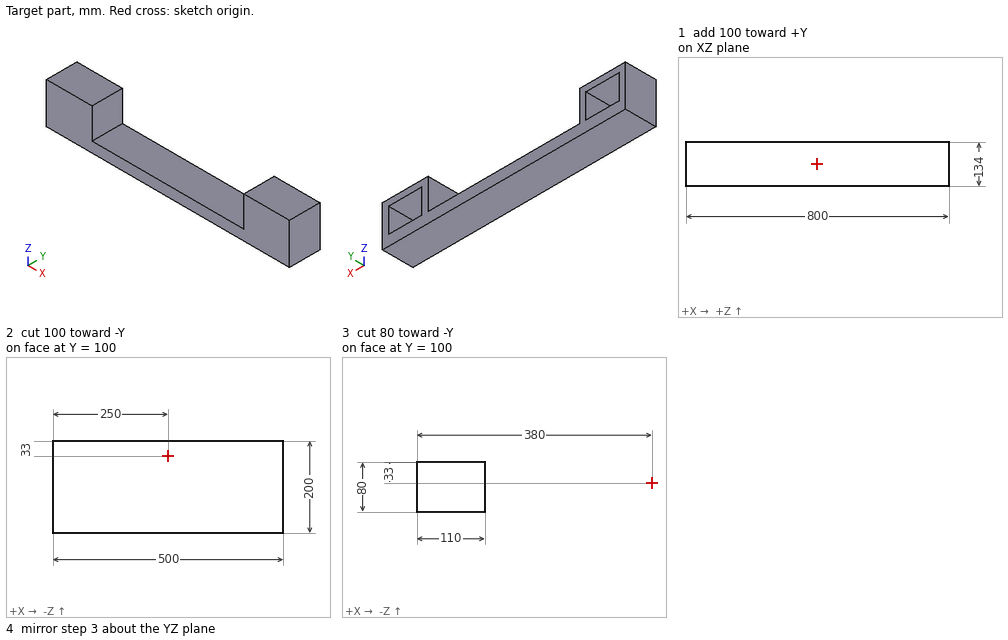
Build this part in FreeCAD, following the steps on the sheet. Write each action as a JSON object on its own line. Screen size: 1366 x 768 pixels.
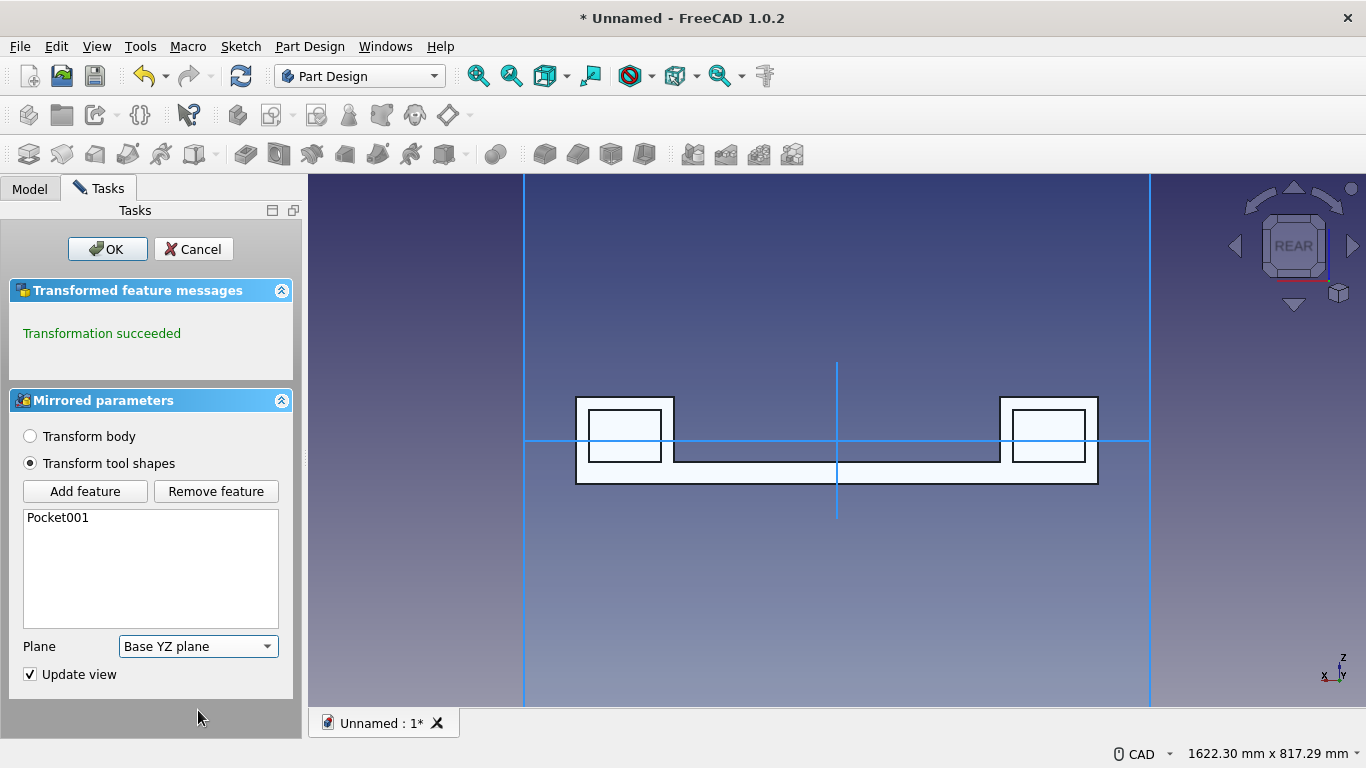
{"action": "left_click", "coordinate": [108, 249]}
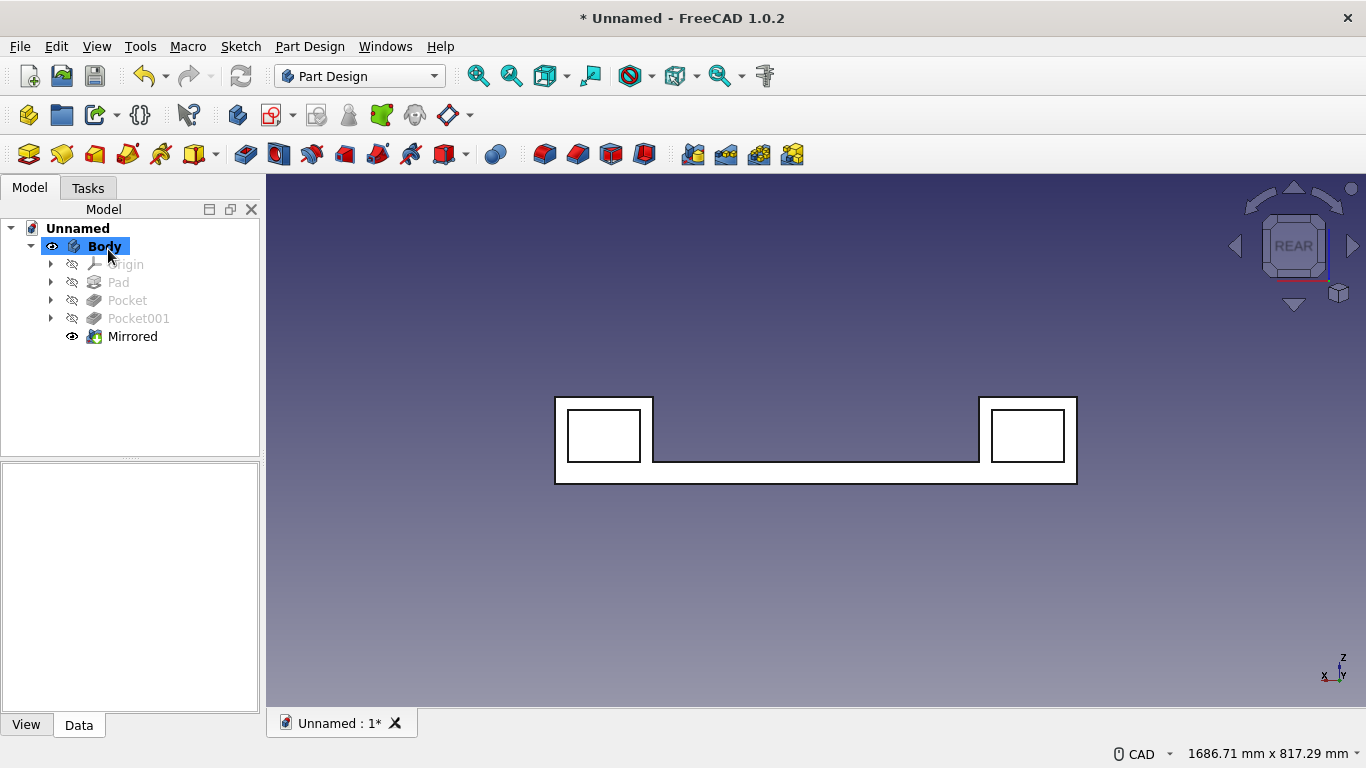
{"action": "key", "text": "0"}